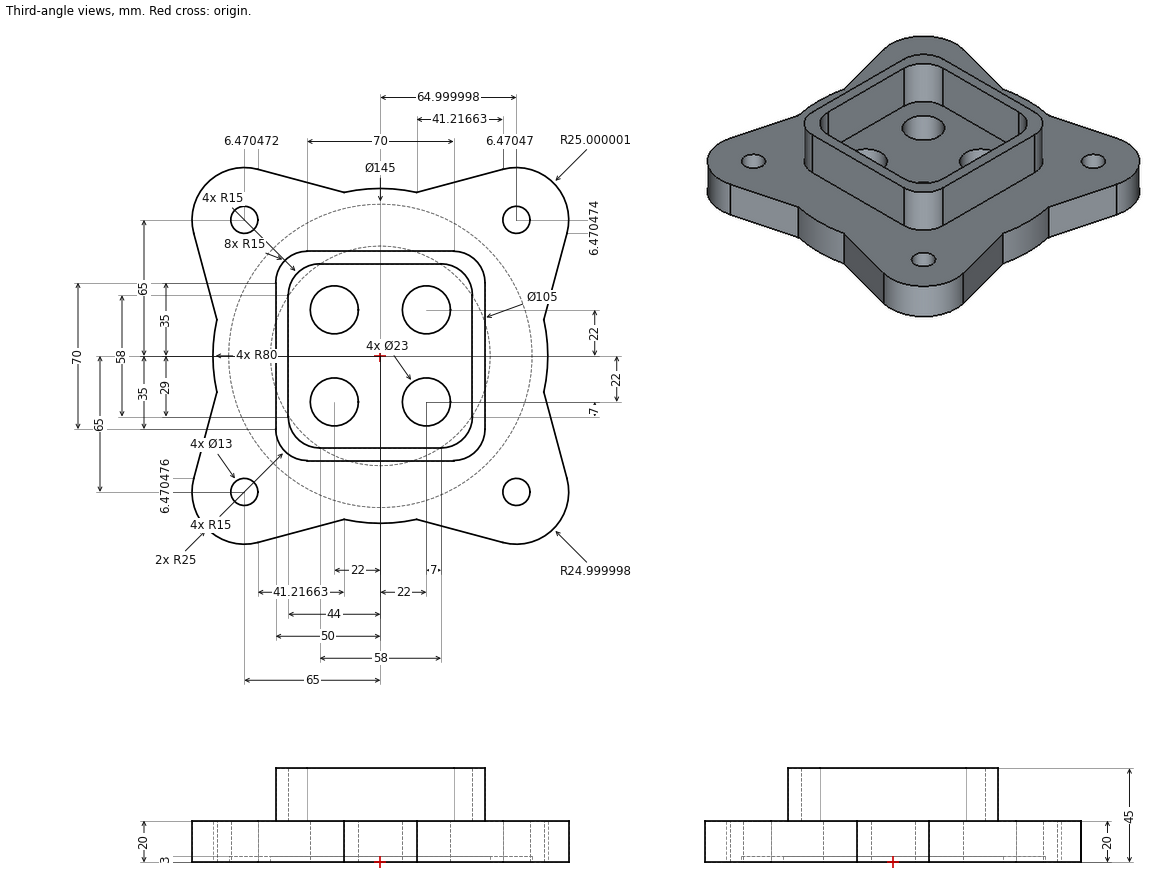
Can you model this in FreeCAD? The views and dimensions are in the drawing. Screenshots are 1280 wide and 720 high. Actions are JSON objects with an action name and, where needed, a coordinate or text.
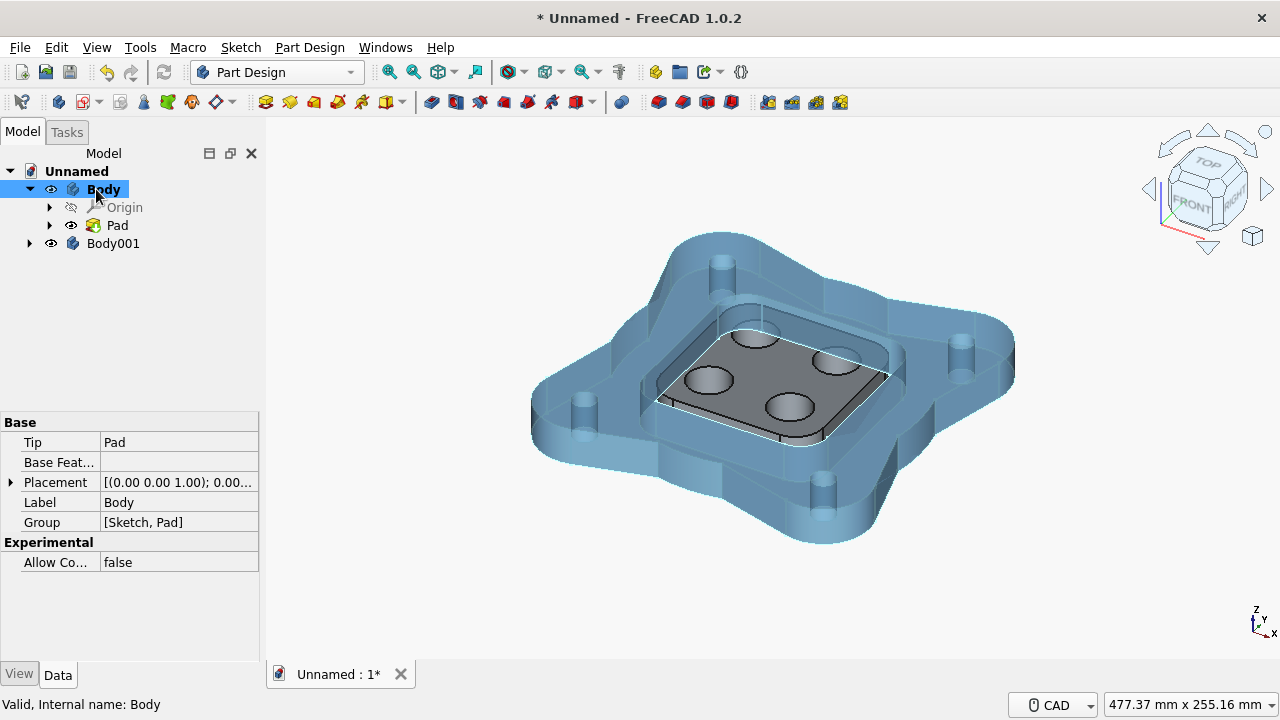
{"action": "left_click", "coordinate": [96, 189]}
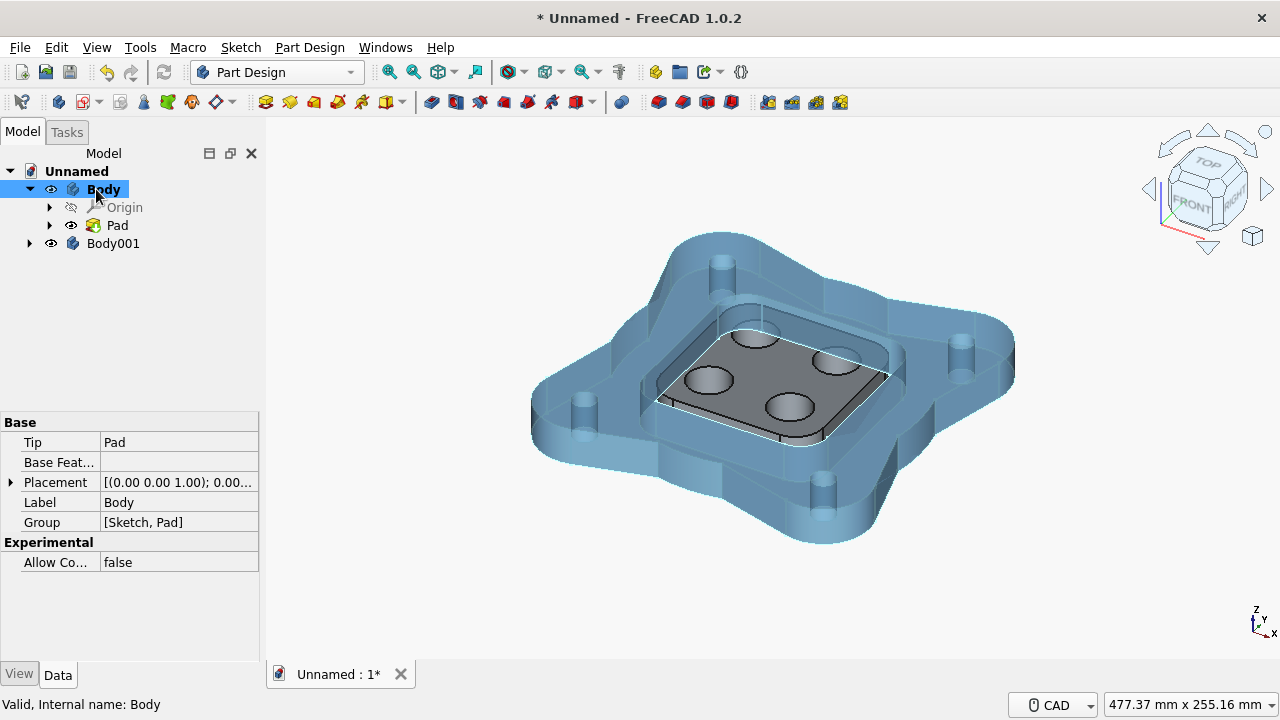
{"action": "left_click", "coordinate": [146, 562]}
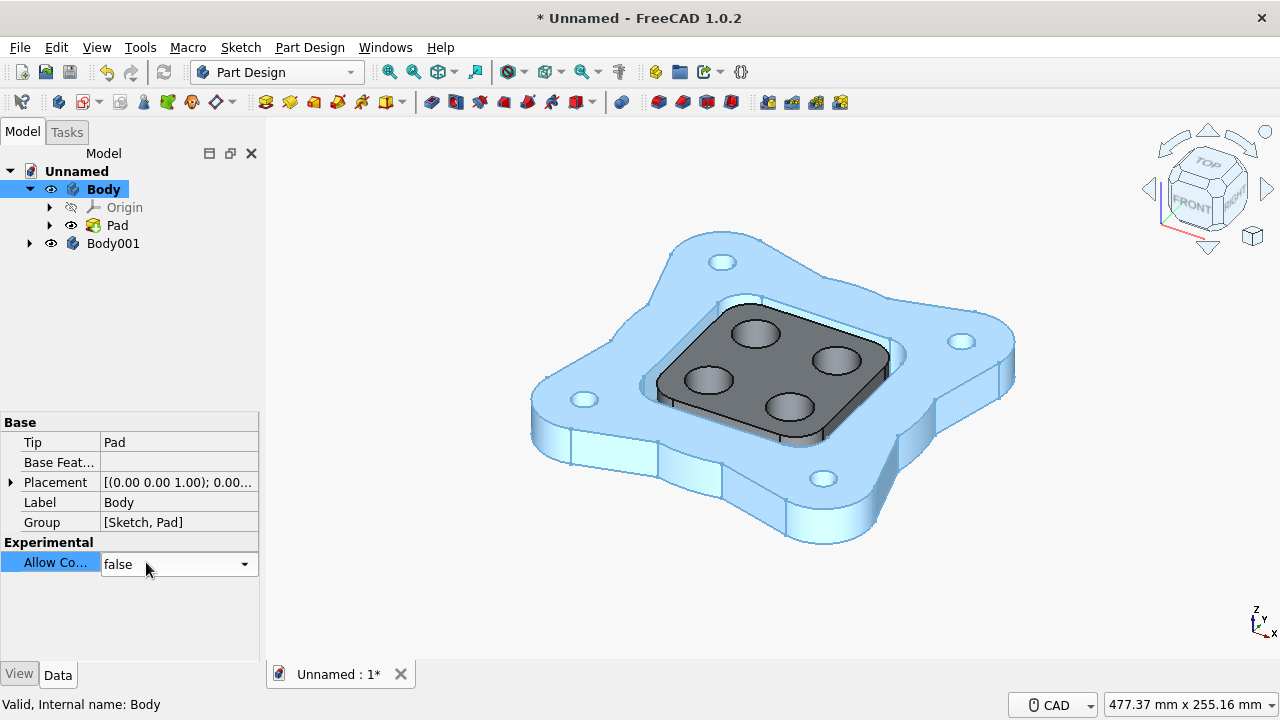
{"action": "left_click", "coordinate": [146, 562]}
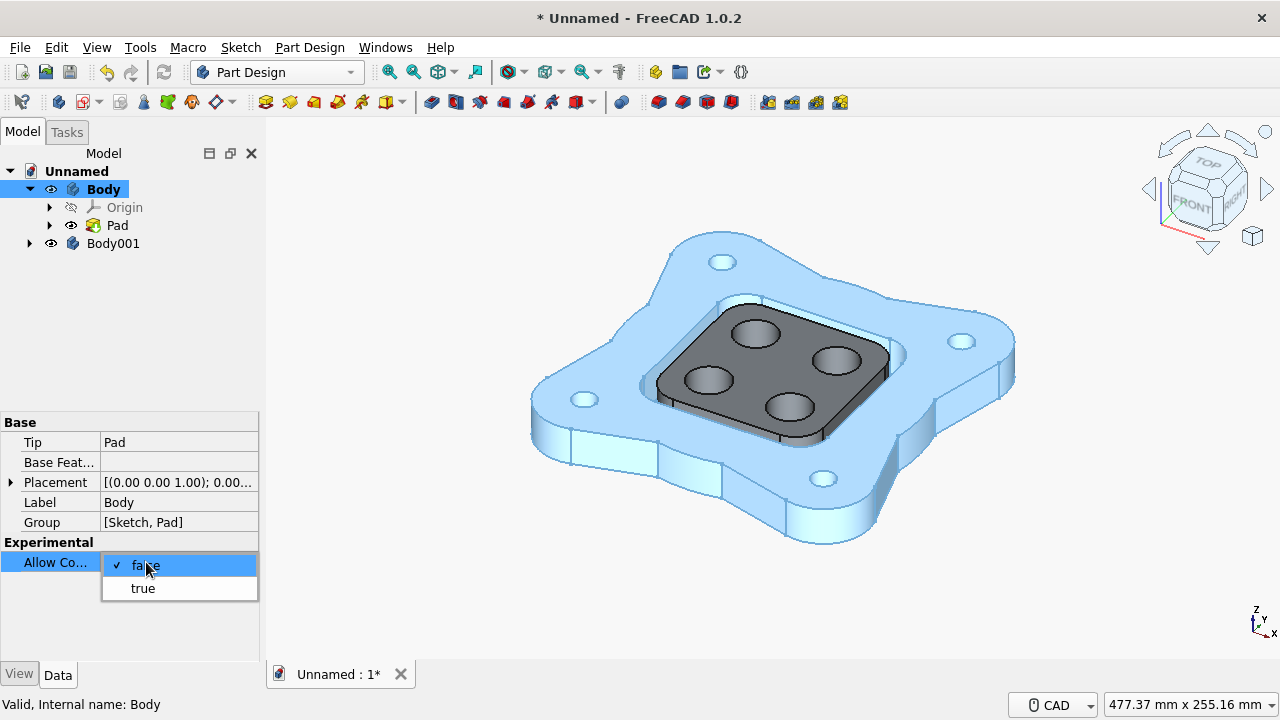
{"action": "left_click", "coordinate": [179, 588]}
{"action": "key", "text": "Return"}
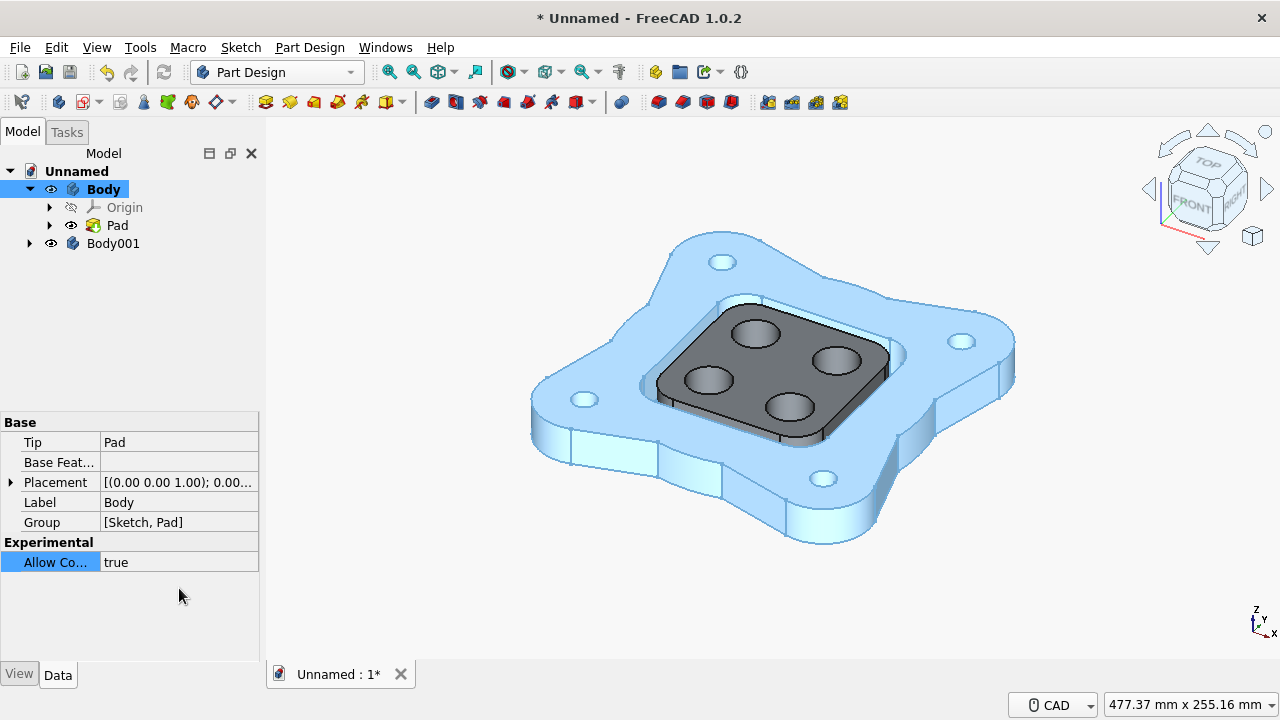
{"action": "left_click", "coordinate": [96, 243]}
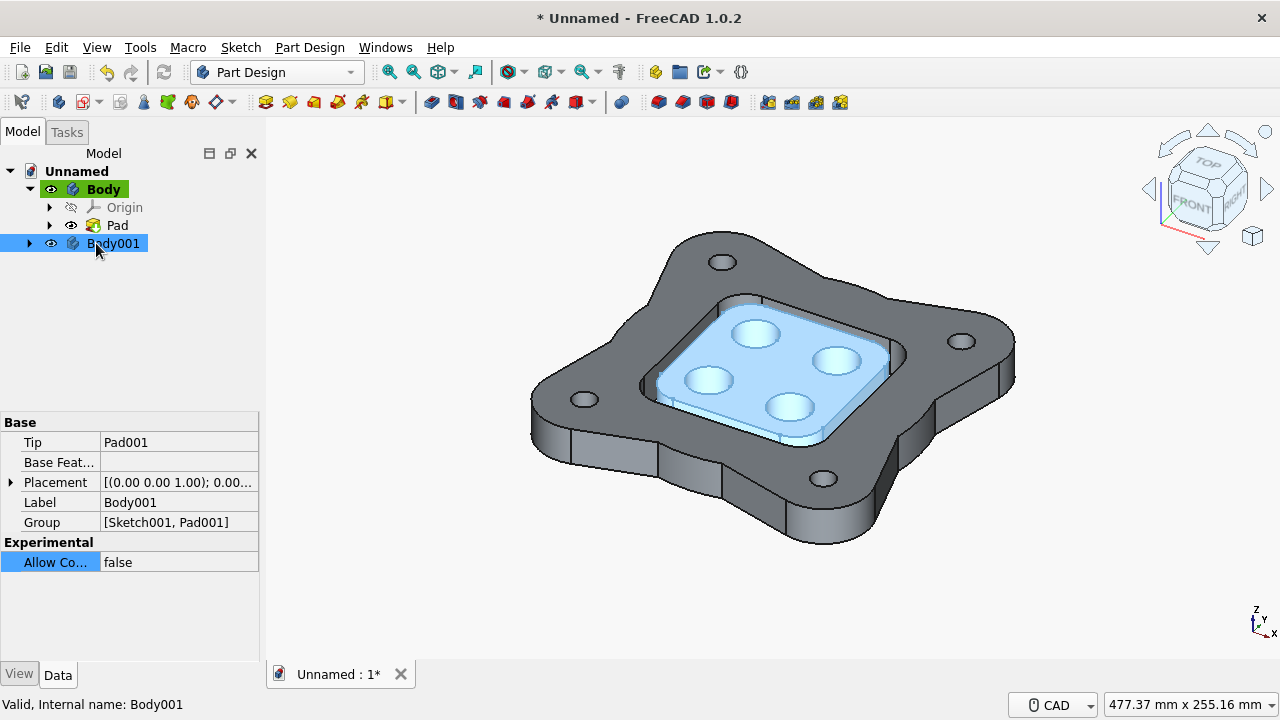
{"action": "left_click", "coordinate": [622, 102]}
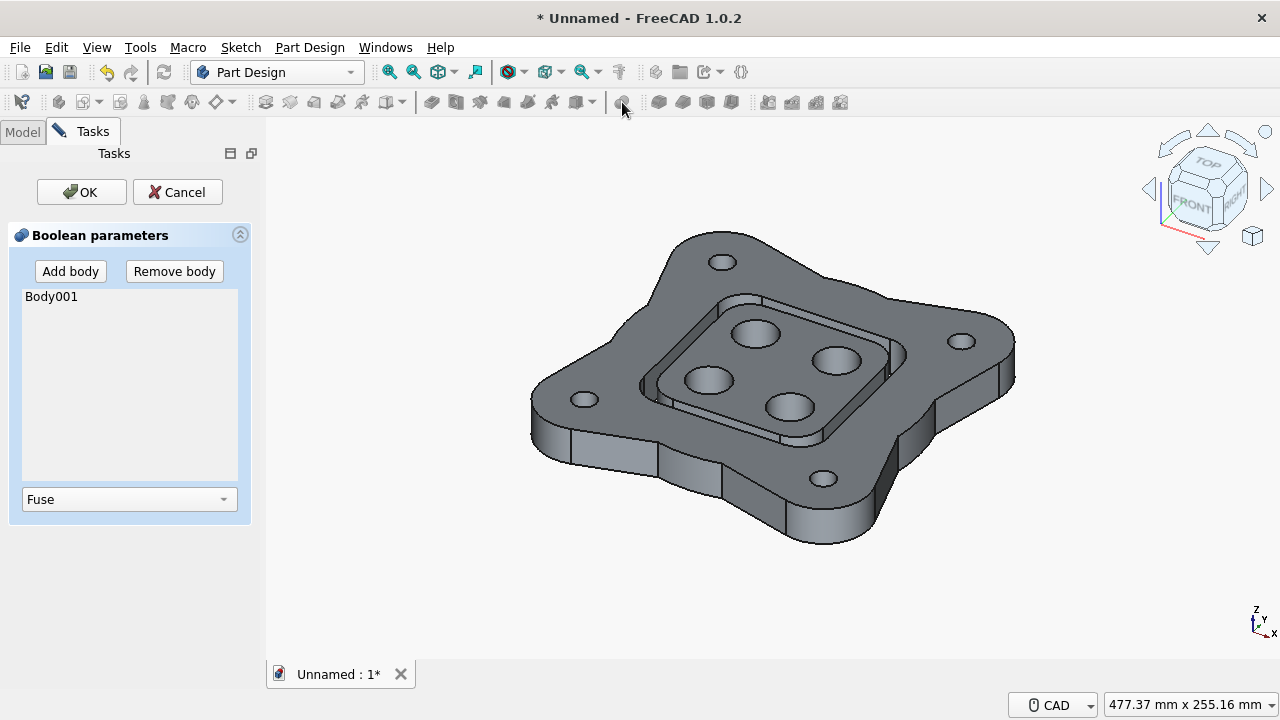
{"action": "left_click", "coordinate": [82, 192]}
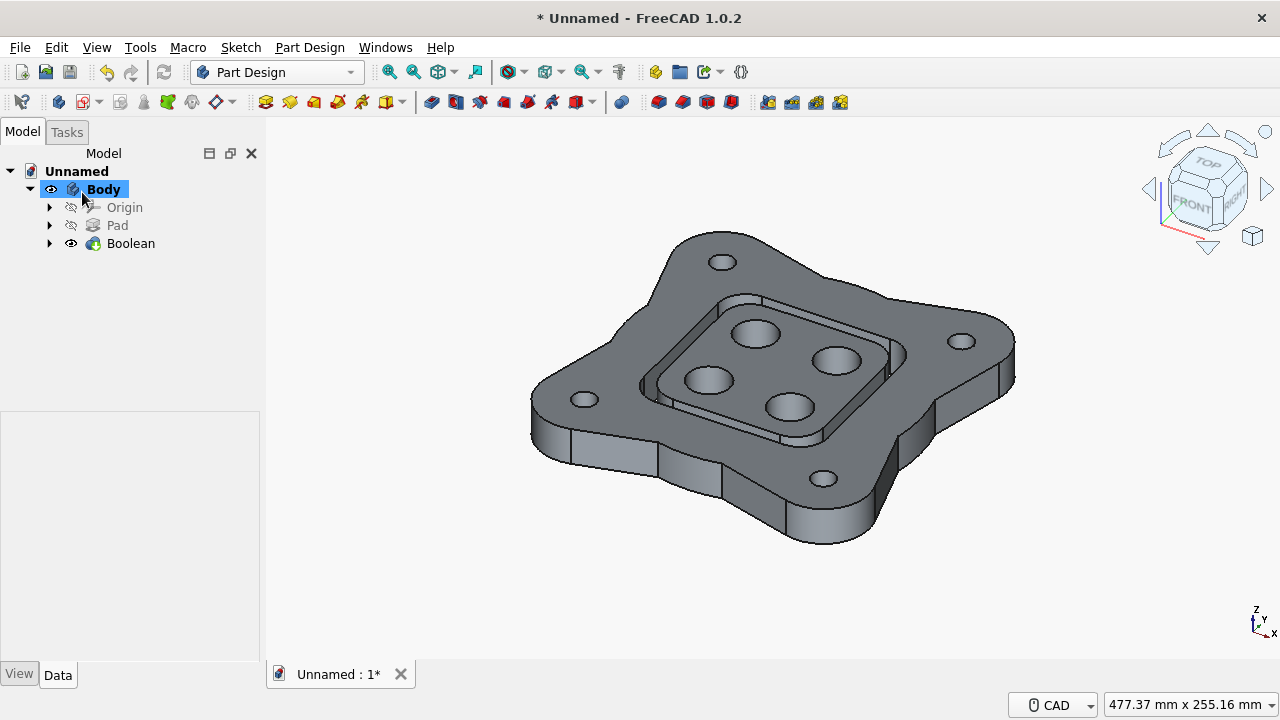
{"action": "key", "text": "5"}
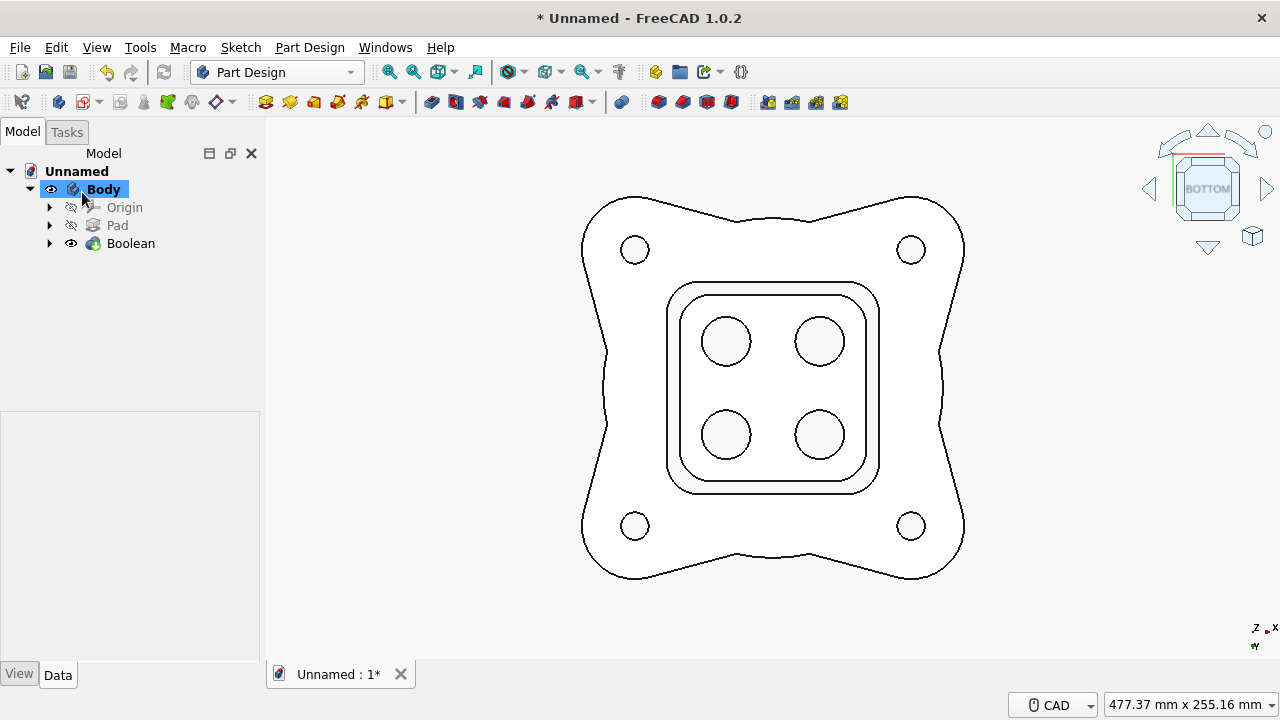
{"action": "left_click", "coordinate": [937, 496]}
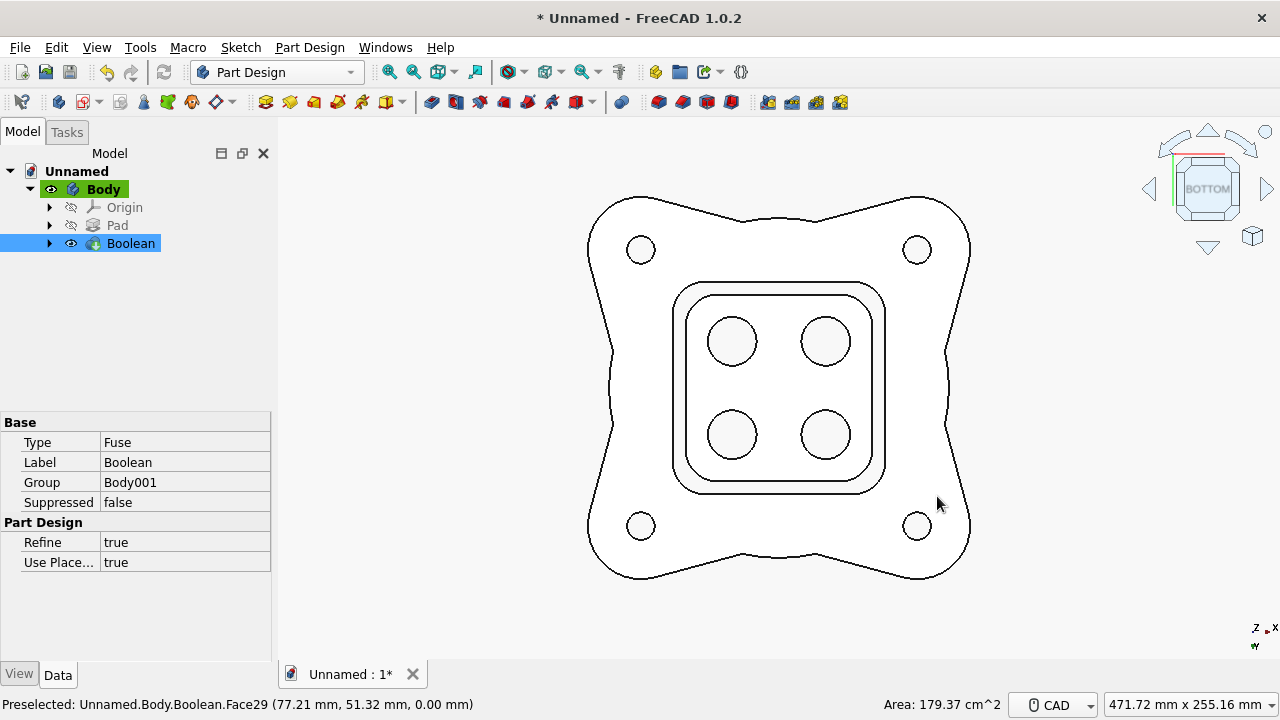
{"action": "left_click", "coordinate": [84, 102]}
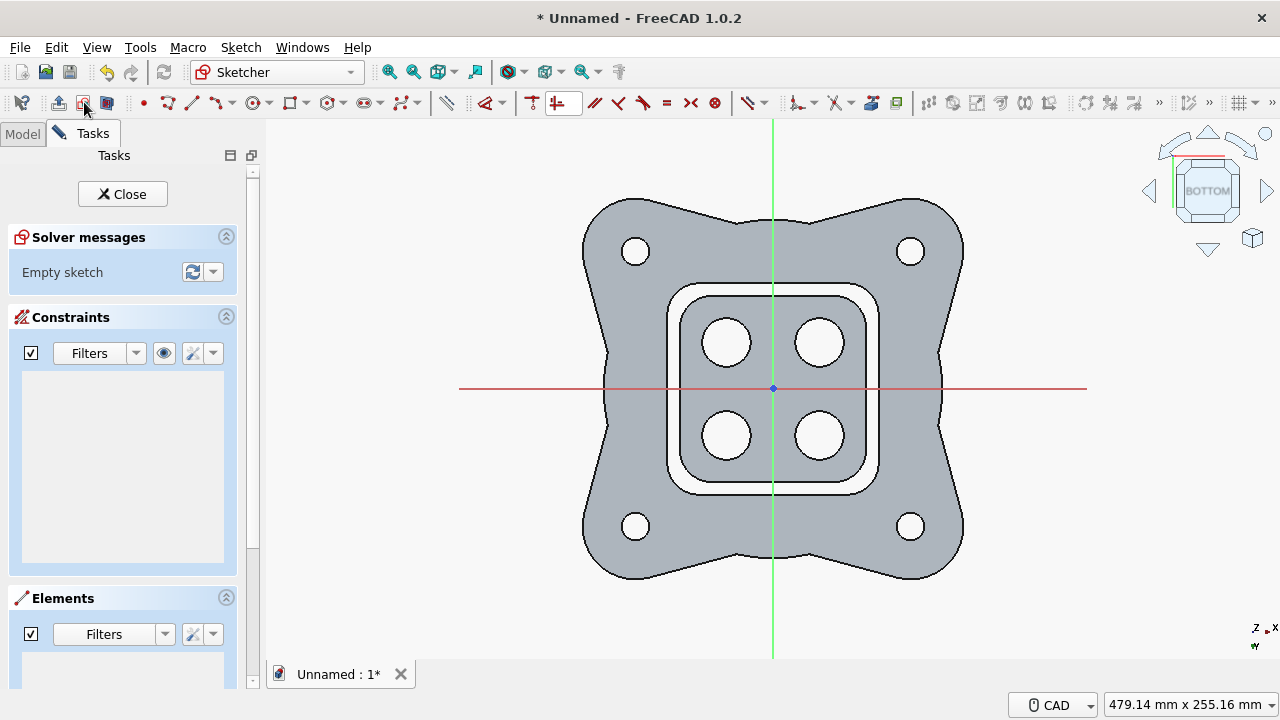
{"action": "scroll", "coordinate": [912, 389], "scroll_direction": "up", "scroll_amount": 2}